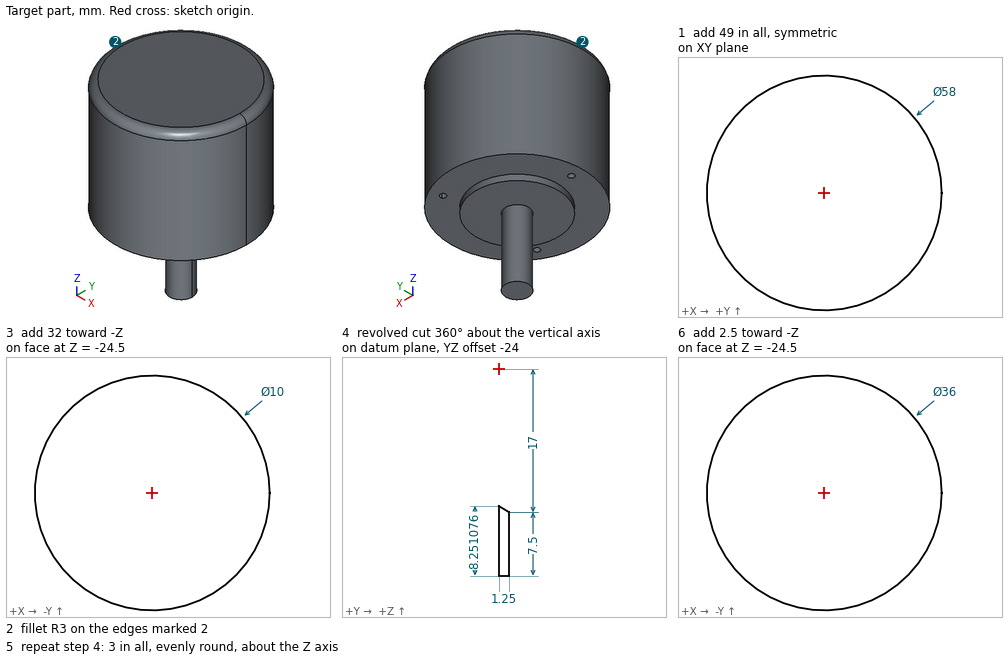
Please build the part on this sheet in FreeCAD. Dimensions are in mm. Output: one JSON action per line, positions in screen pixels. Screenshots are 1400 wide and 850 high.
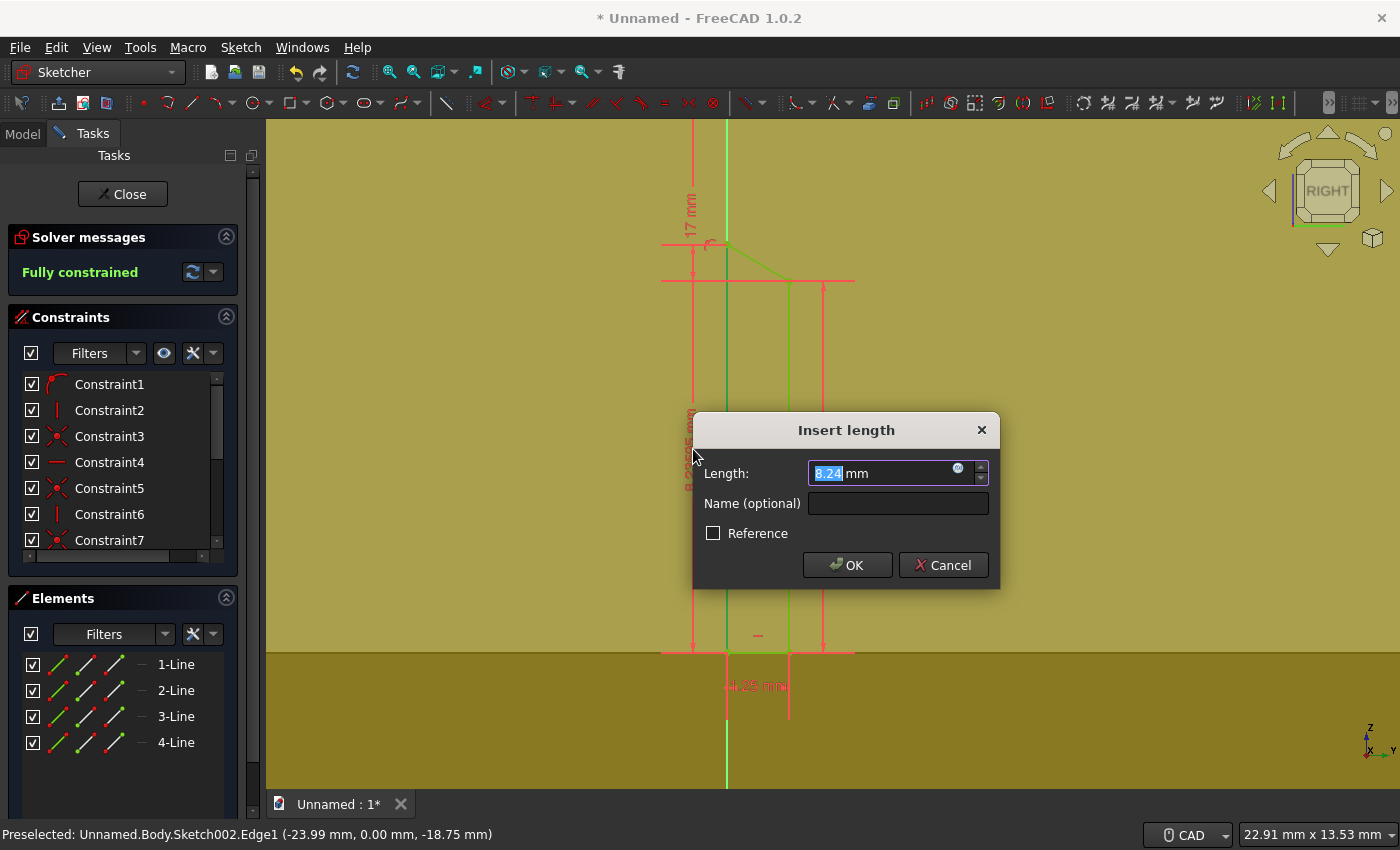
{"action": "type", "text": "8.251076"}
{"action": "key", "text": "Return"}
{"action": "key", "text": "Escape"}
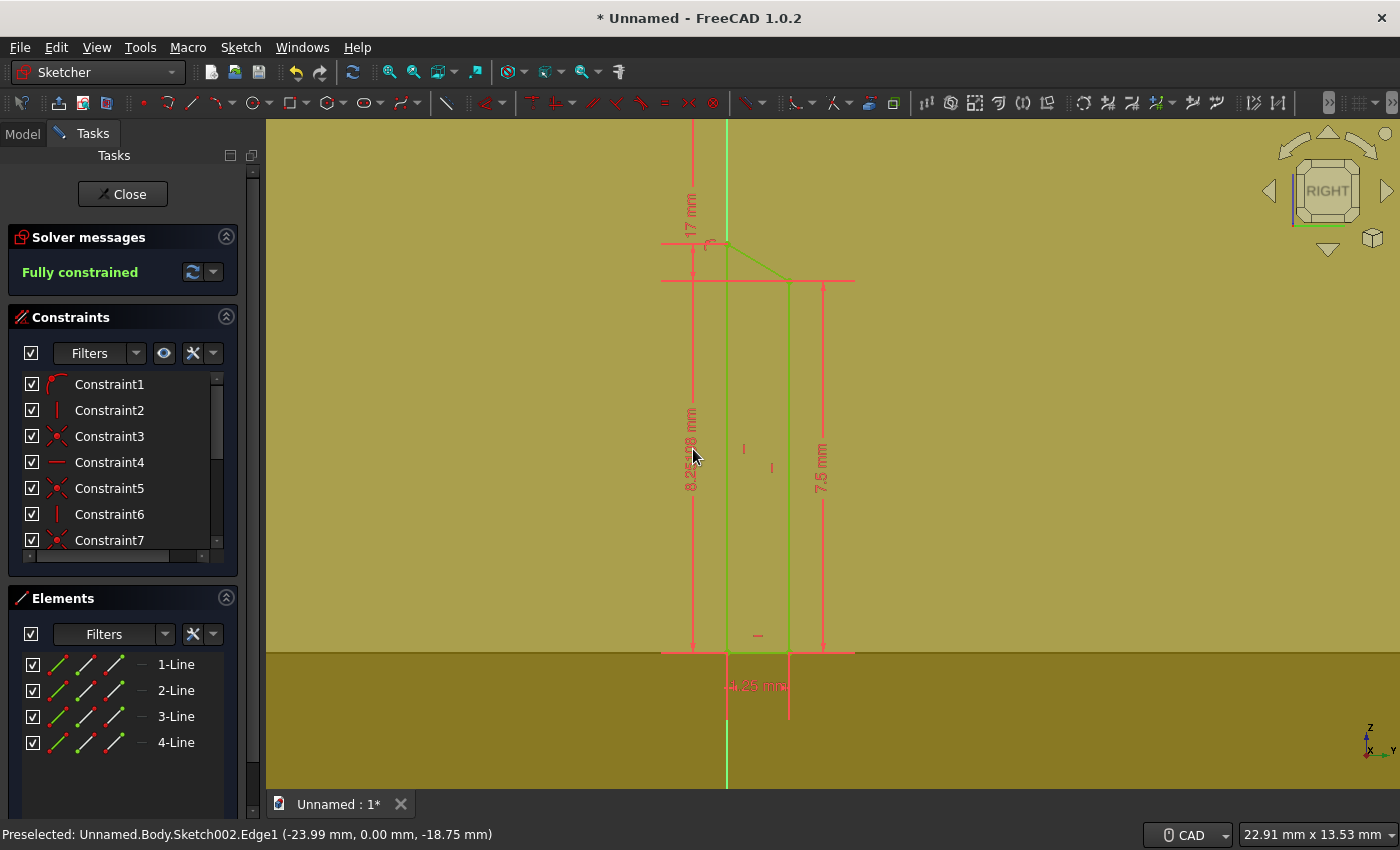
{"action": "left_click", "coordinate": [123, 194]}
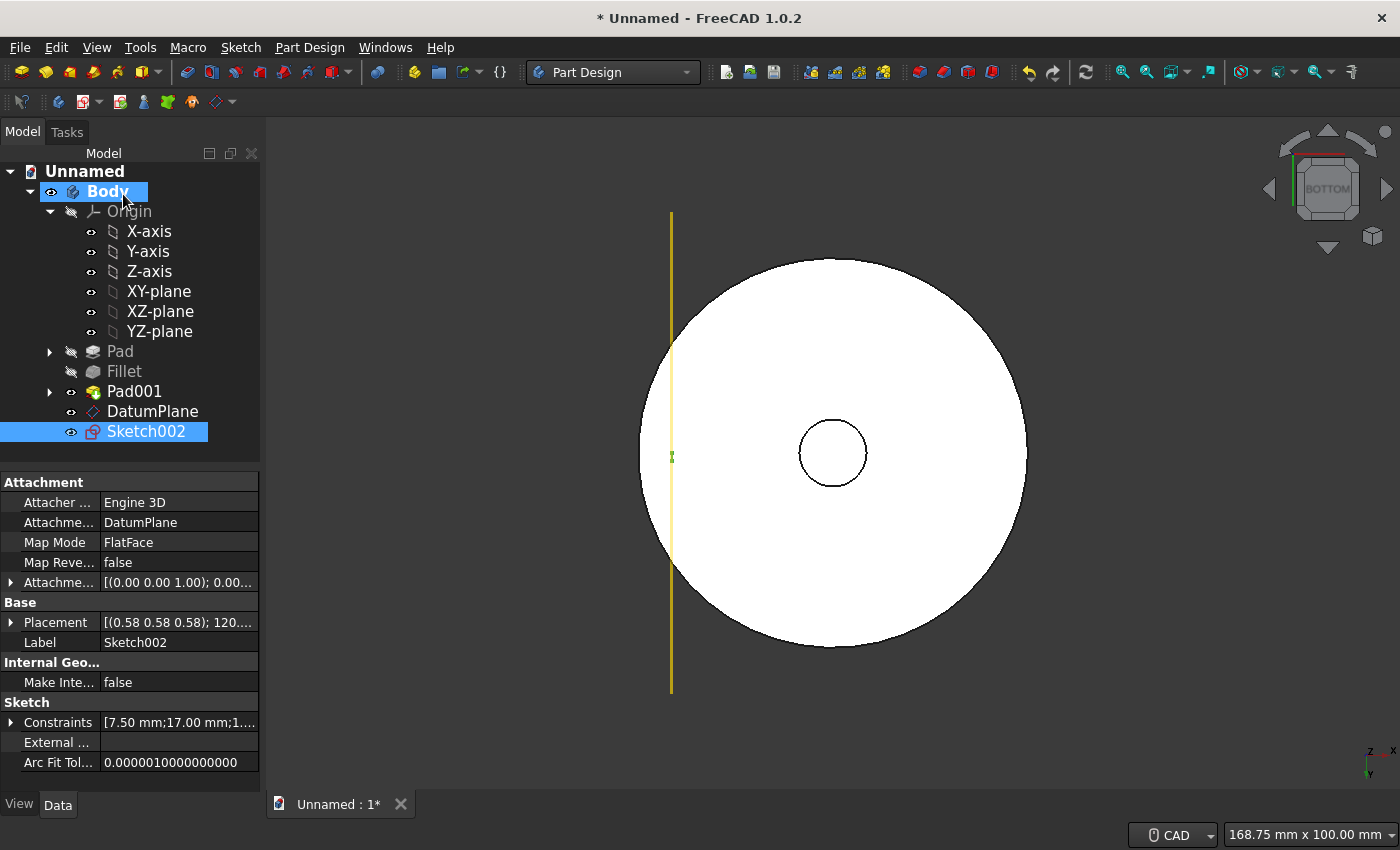
{"action": "left_click", "coordinate": [236, 72]}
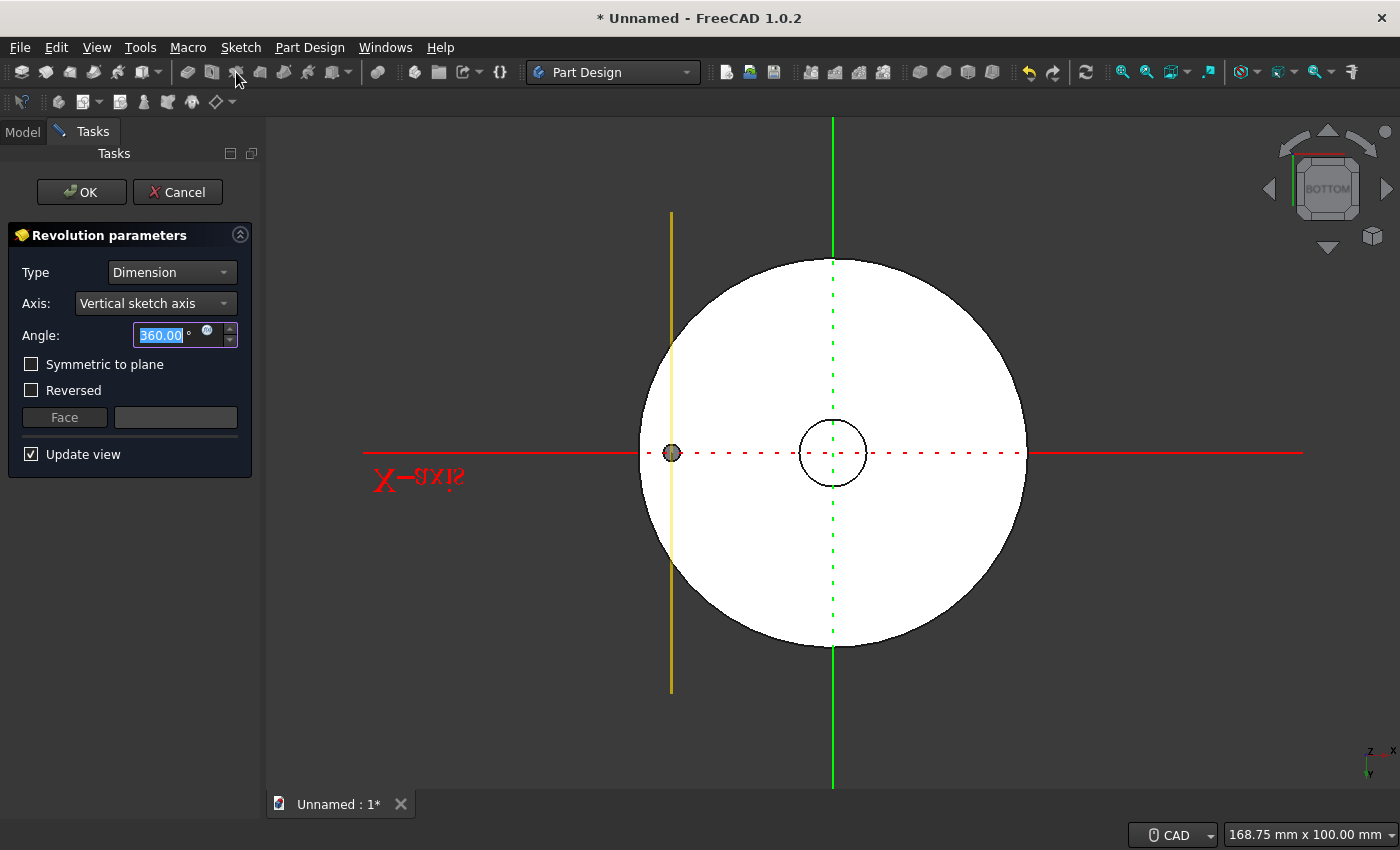
{"action": "left_click", "coordinate": [82, 192]}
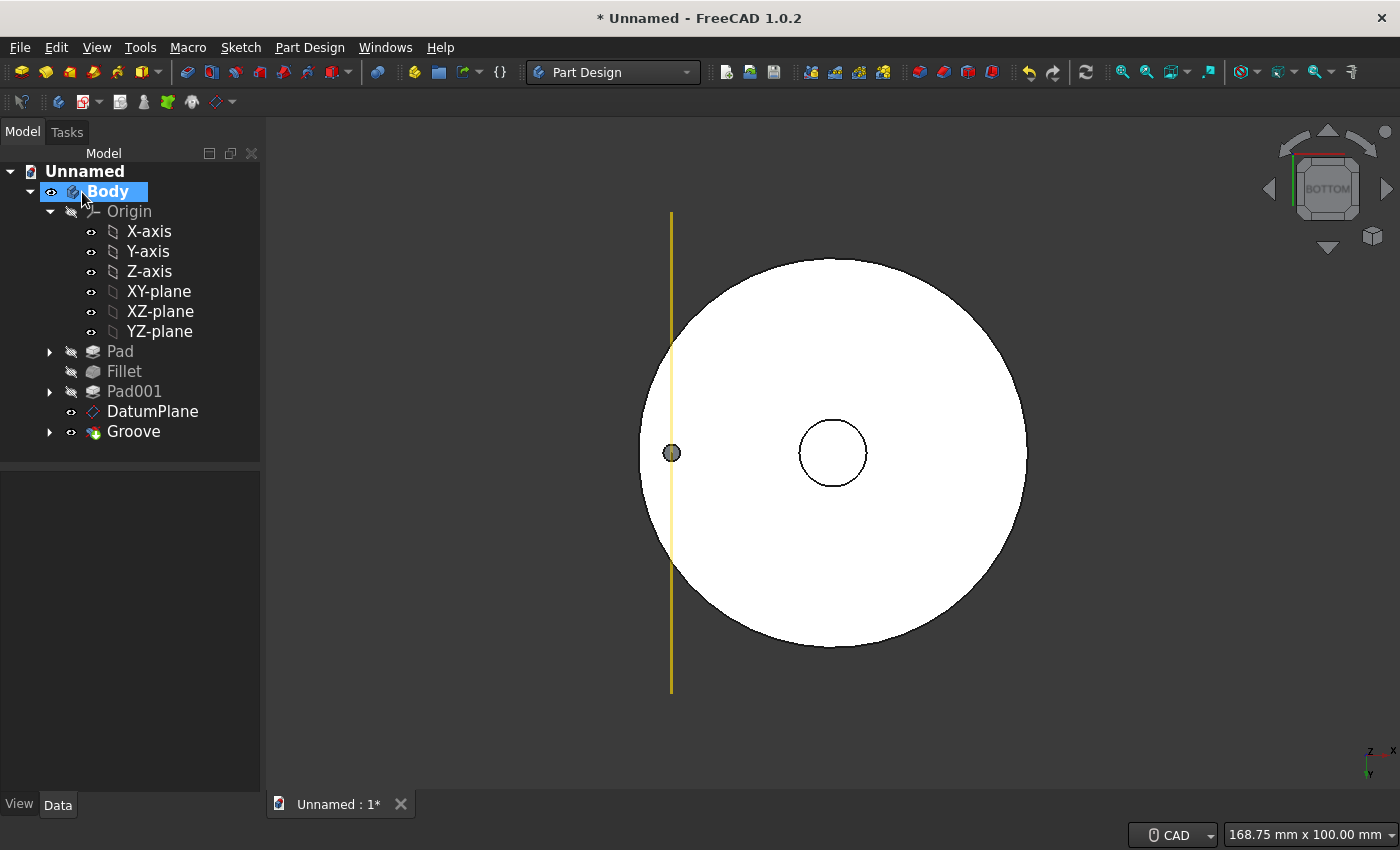
{"action": "left_click", "coordinate": [116, 412]}
{"action": "key", "text": "space"}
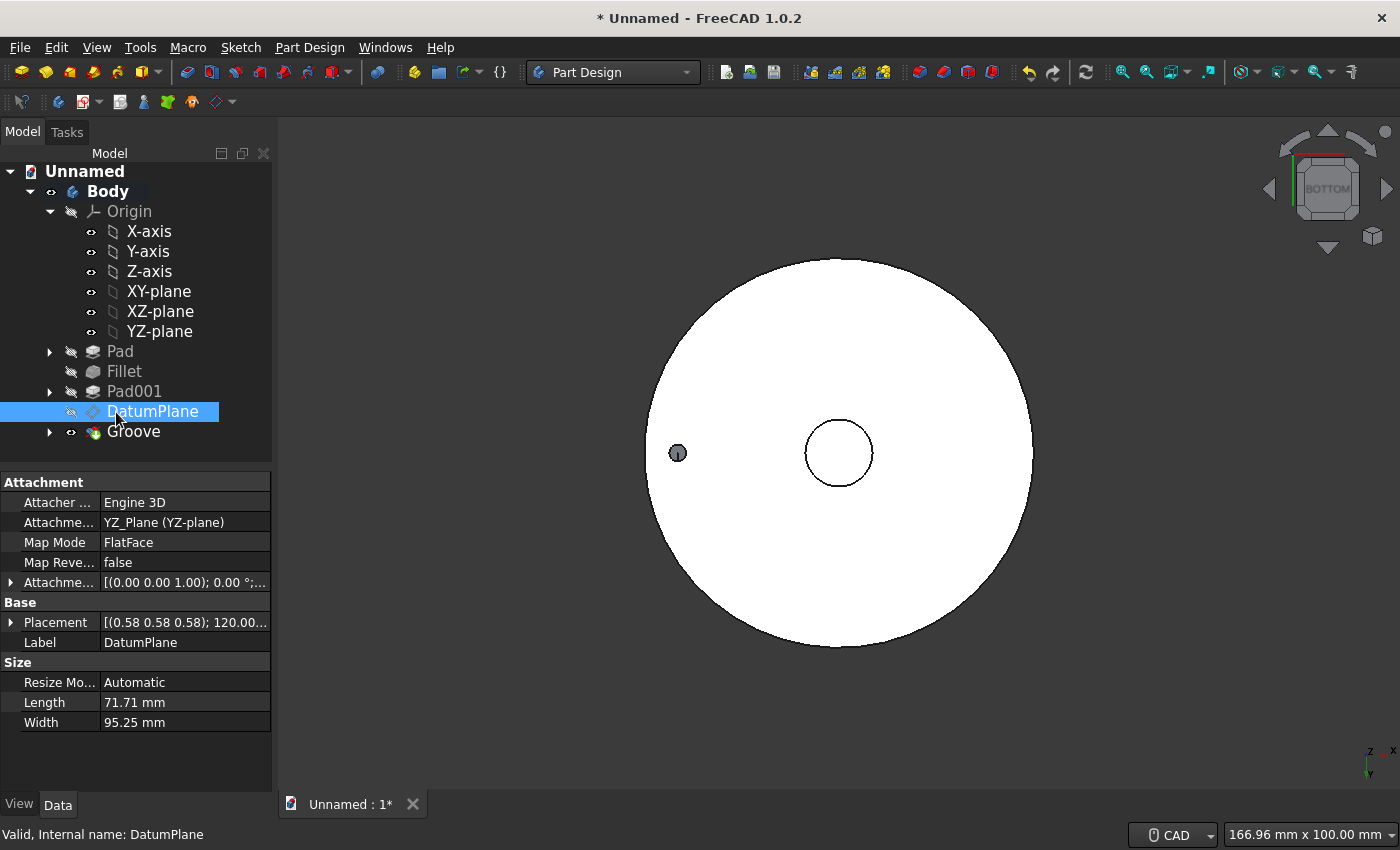
{"action": "left_click", "coordinate": [116, 432]}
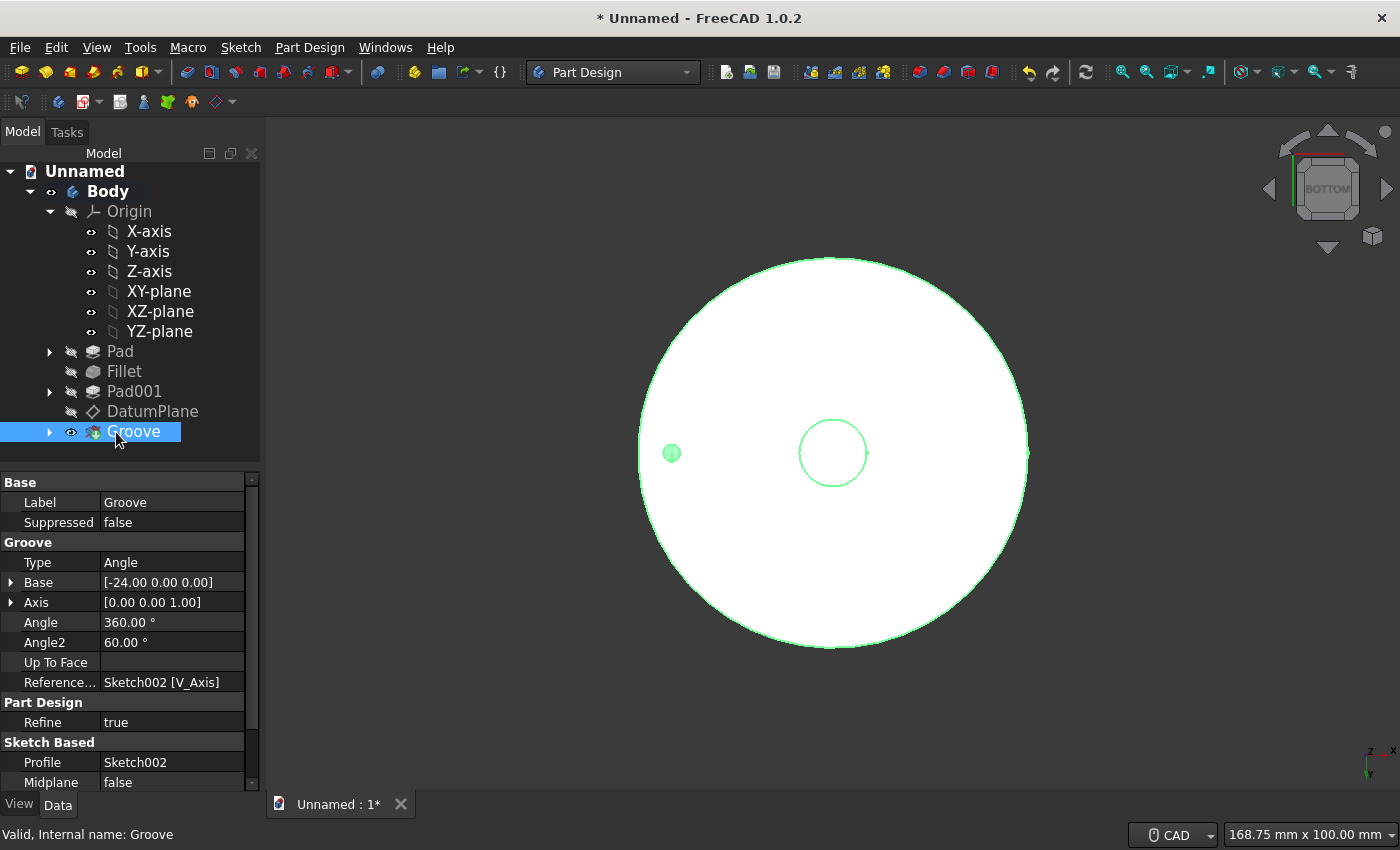
{"action": "left_click", "coordinate": [860, 72]}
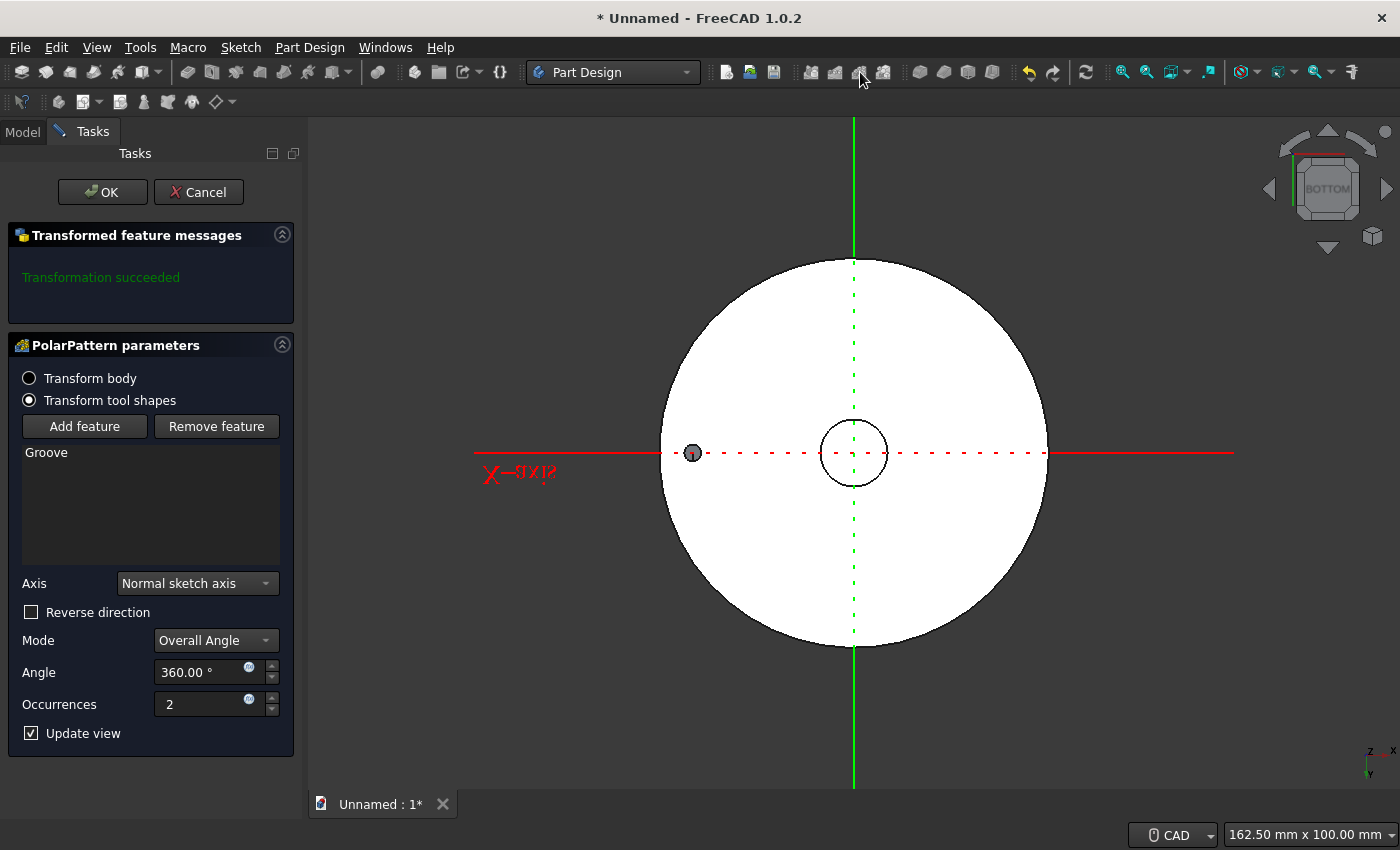
{"action": "left_click", "coordinate": [198, 584]}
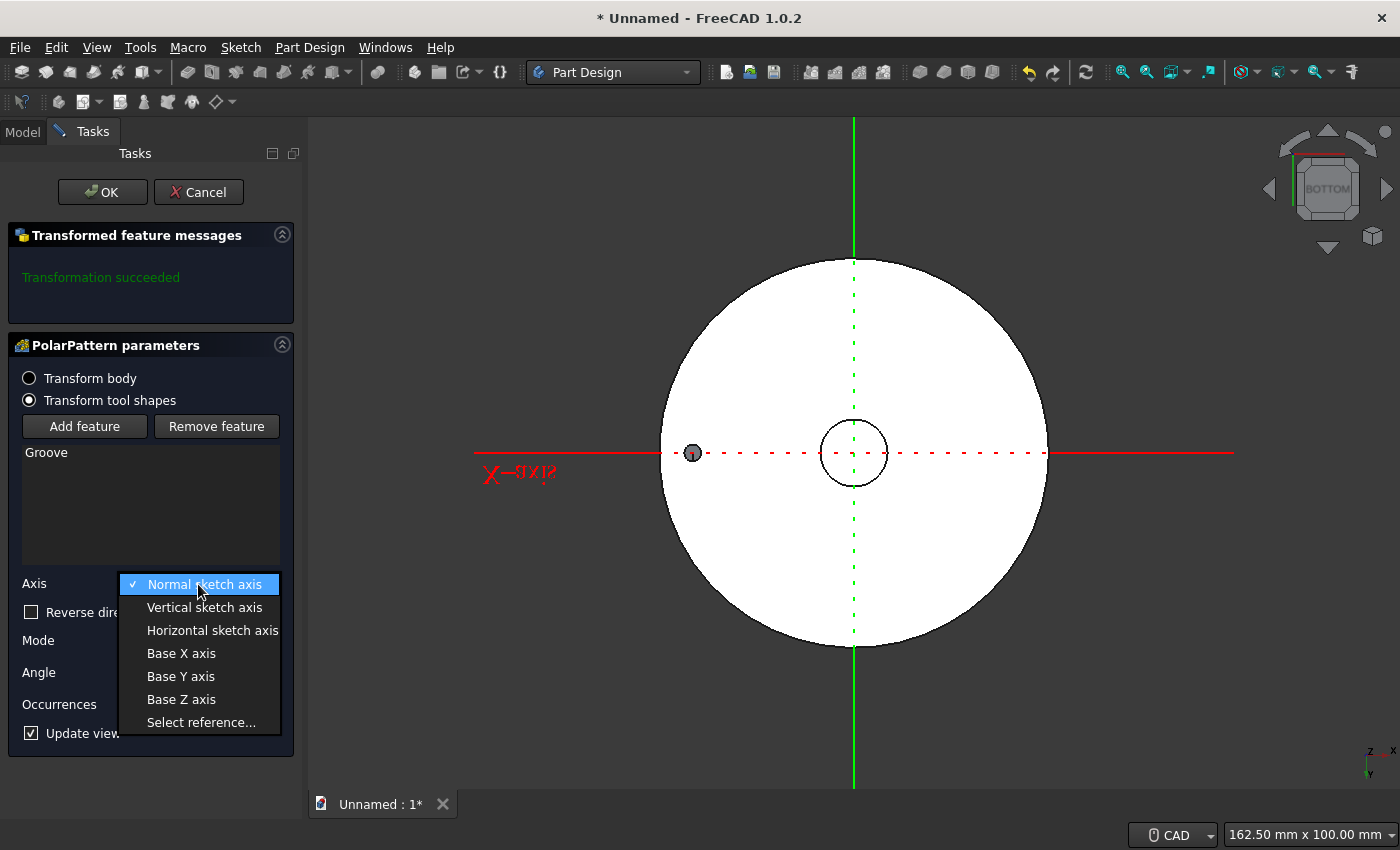
{"action": "left_click", "coordinate": [198, 700]}